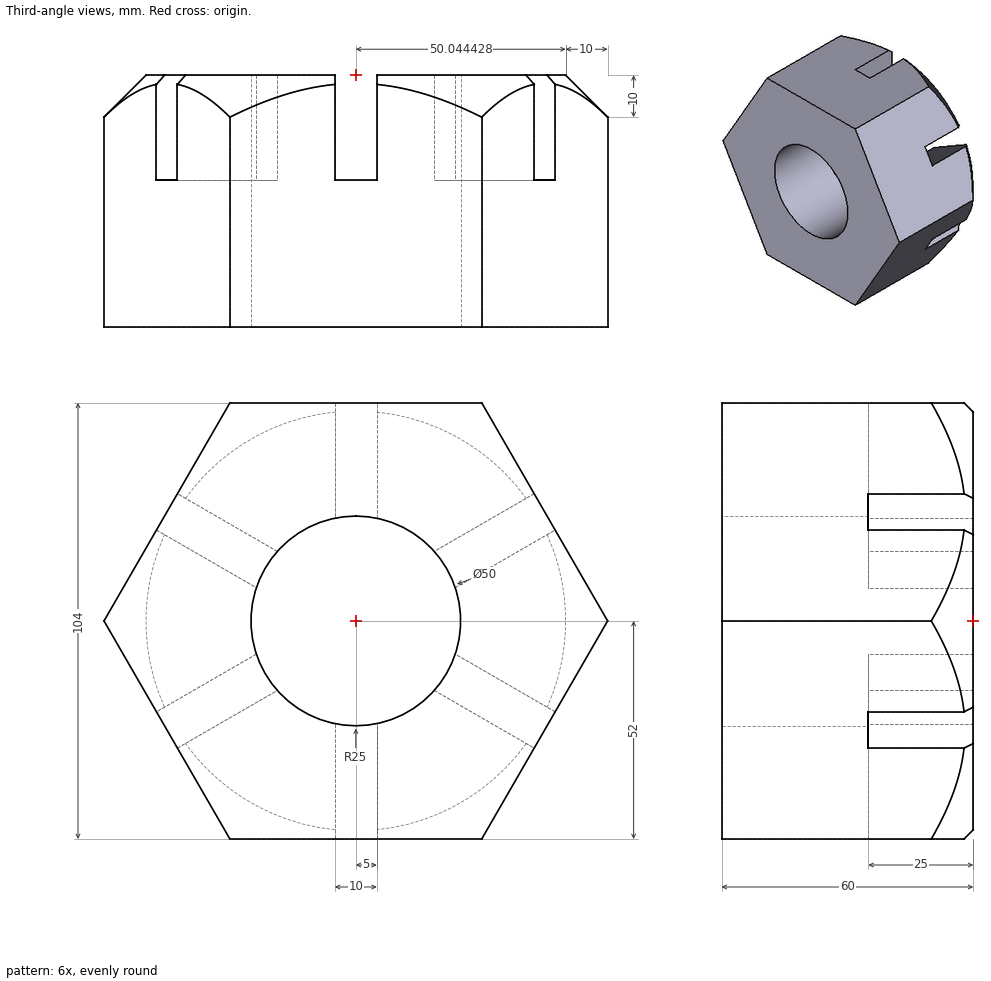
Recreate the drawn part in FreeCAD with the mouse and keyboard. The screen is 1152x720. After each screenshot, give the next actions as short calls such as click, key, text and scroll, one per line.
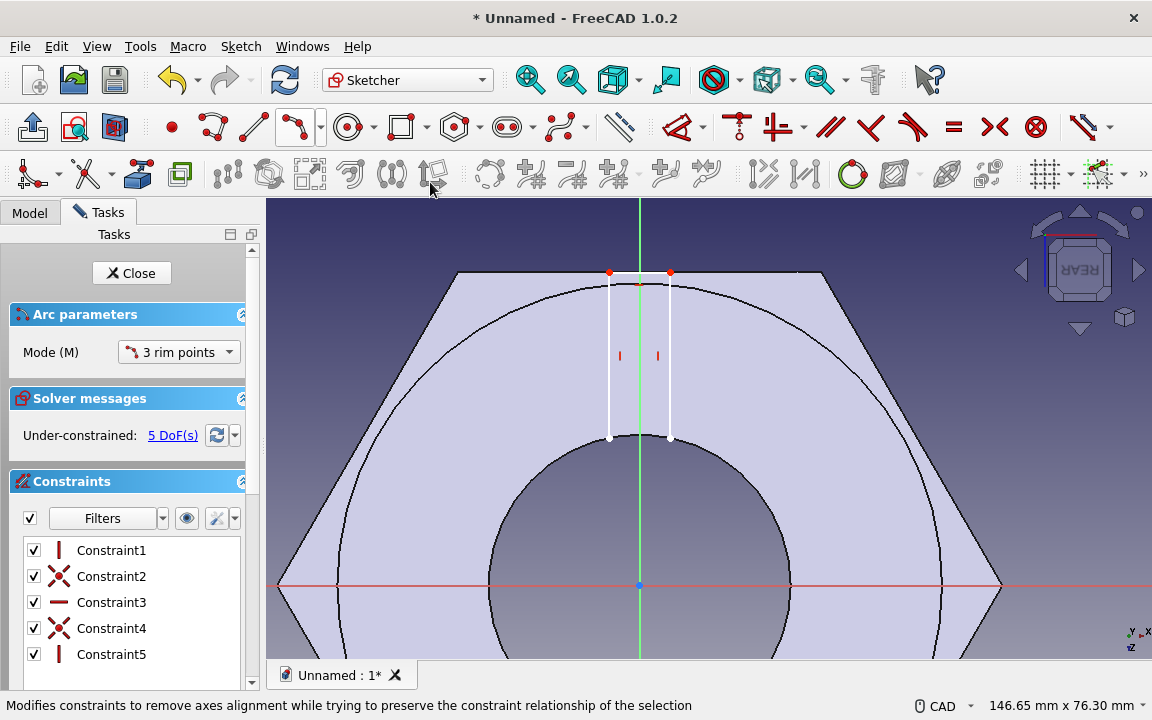
click(609, 439)
click(670, 439)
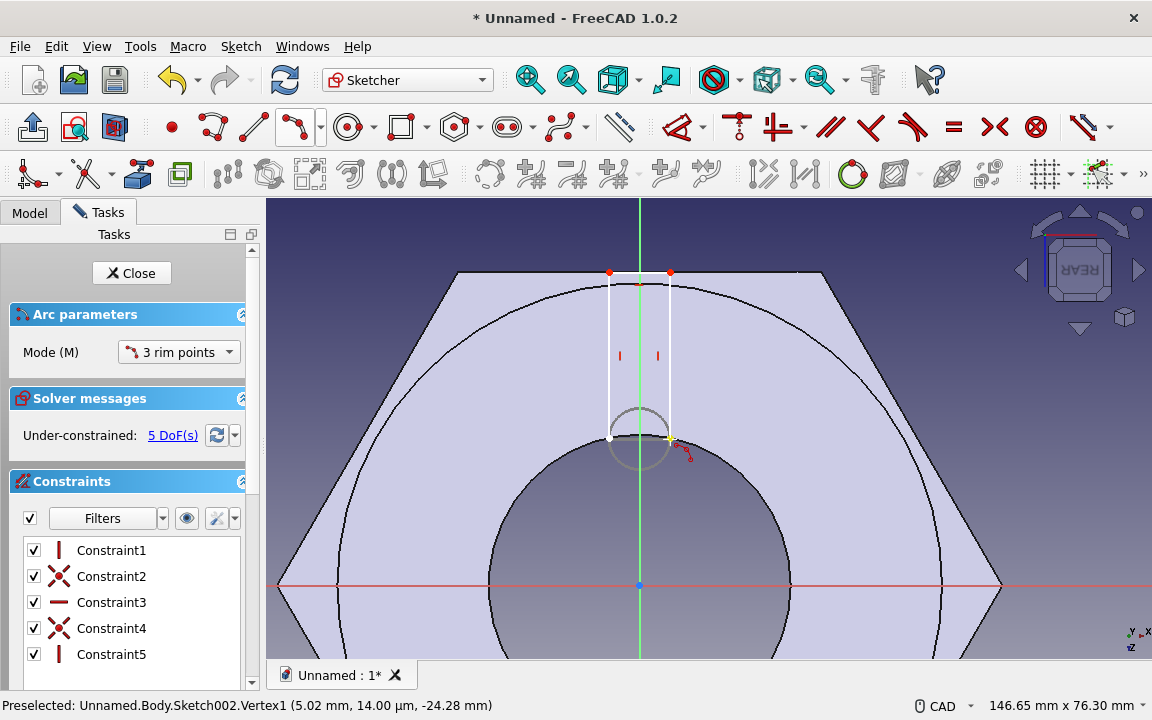
scroll(646, 435, up, 9)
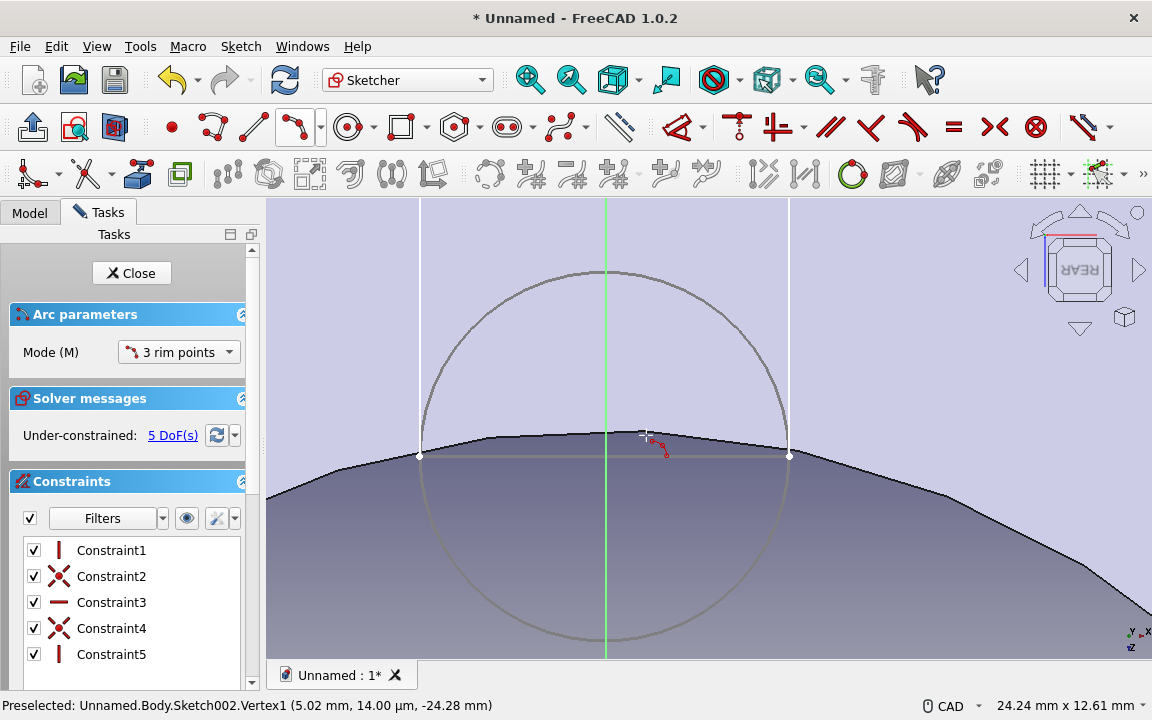
click(642, 431)
key(Escape)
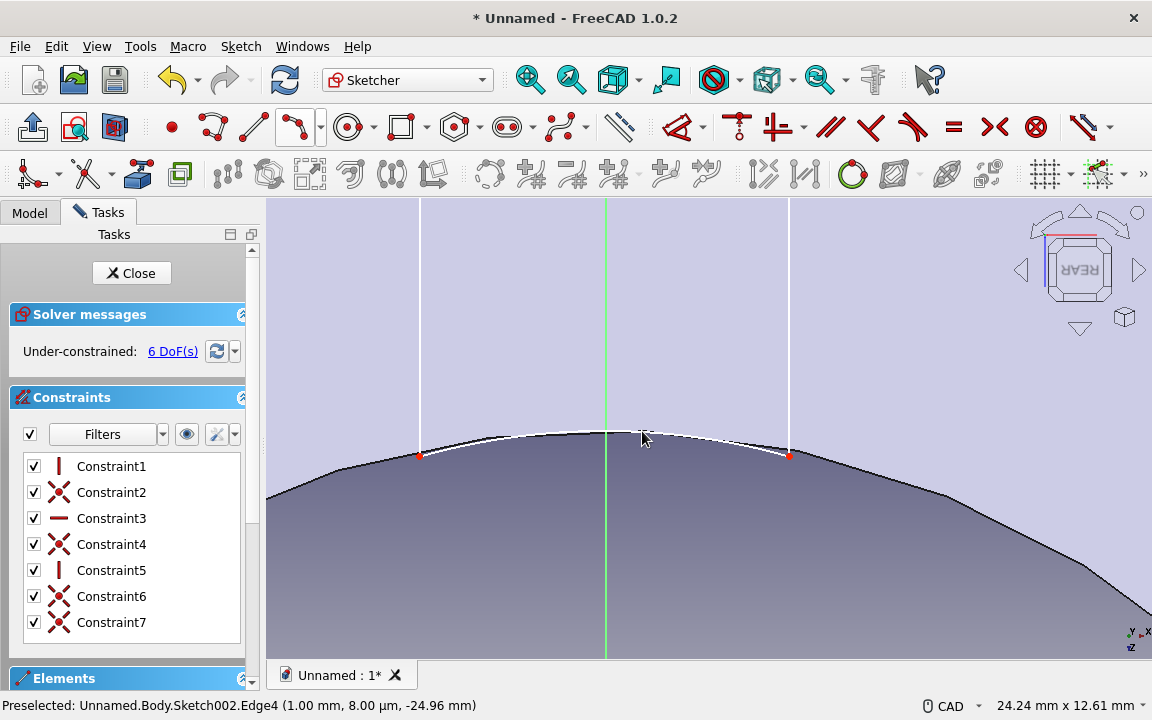
scroll(647, 435, down, 9)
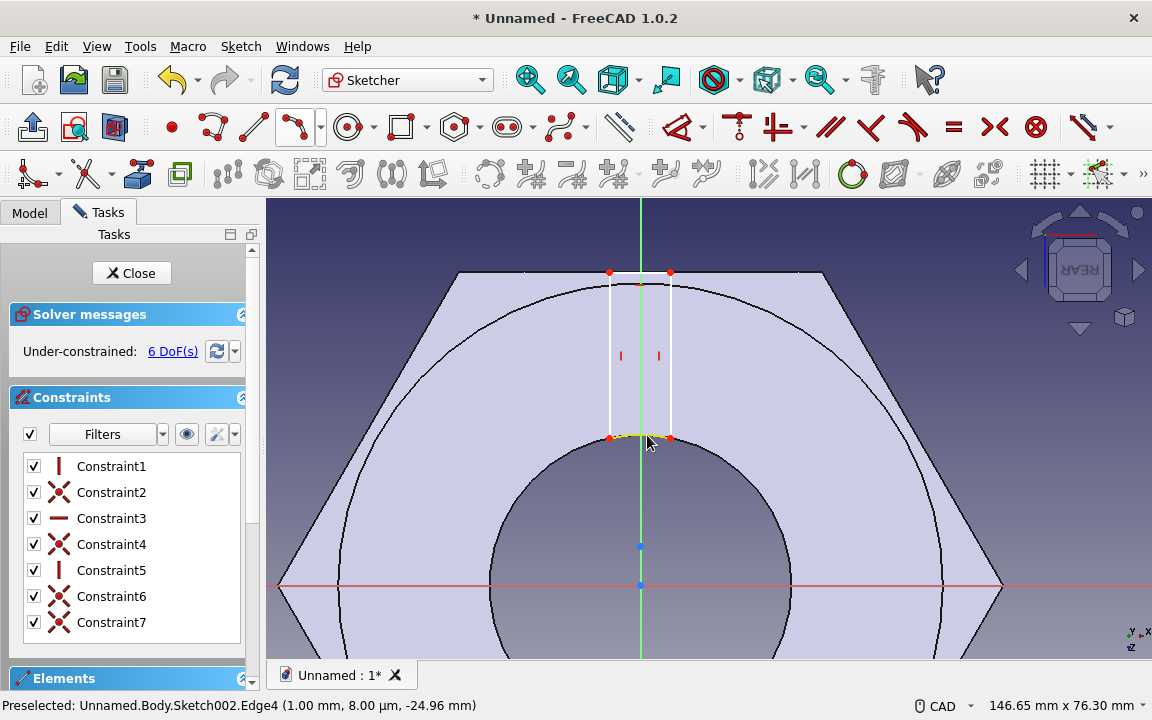
drag(630, 537, 651, 596)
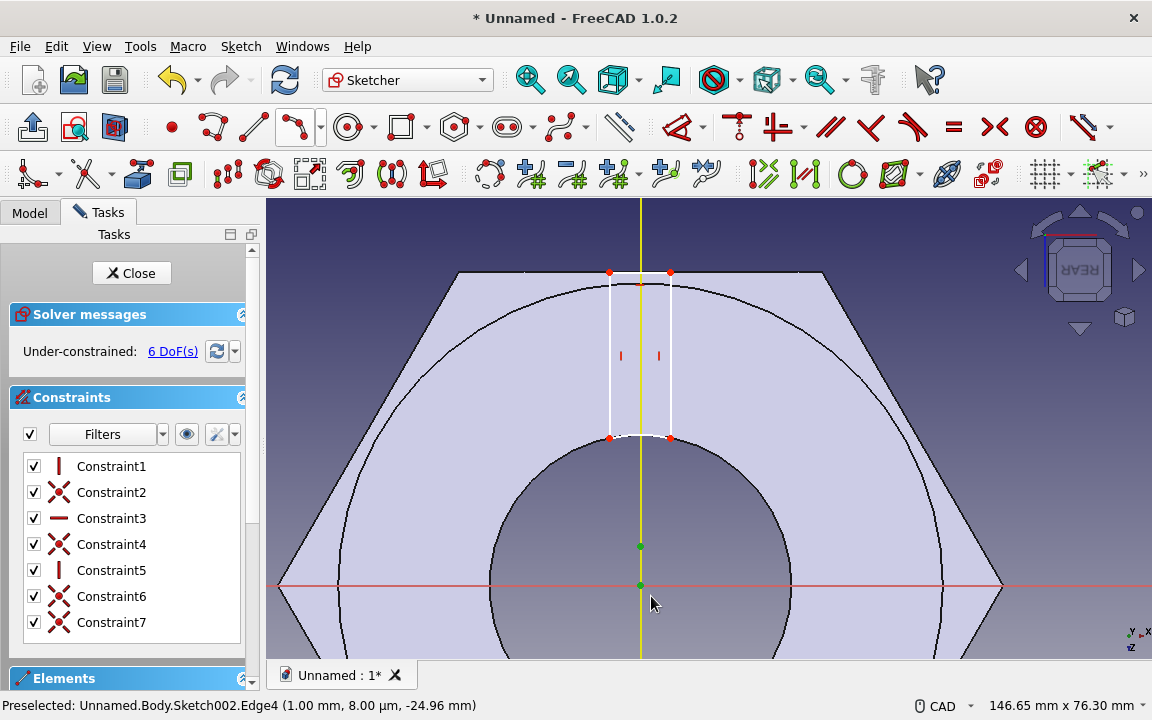
click(737, 128)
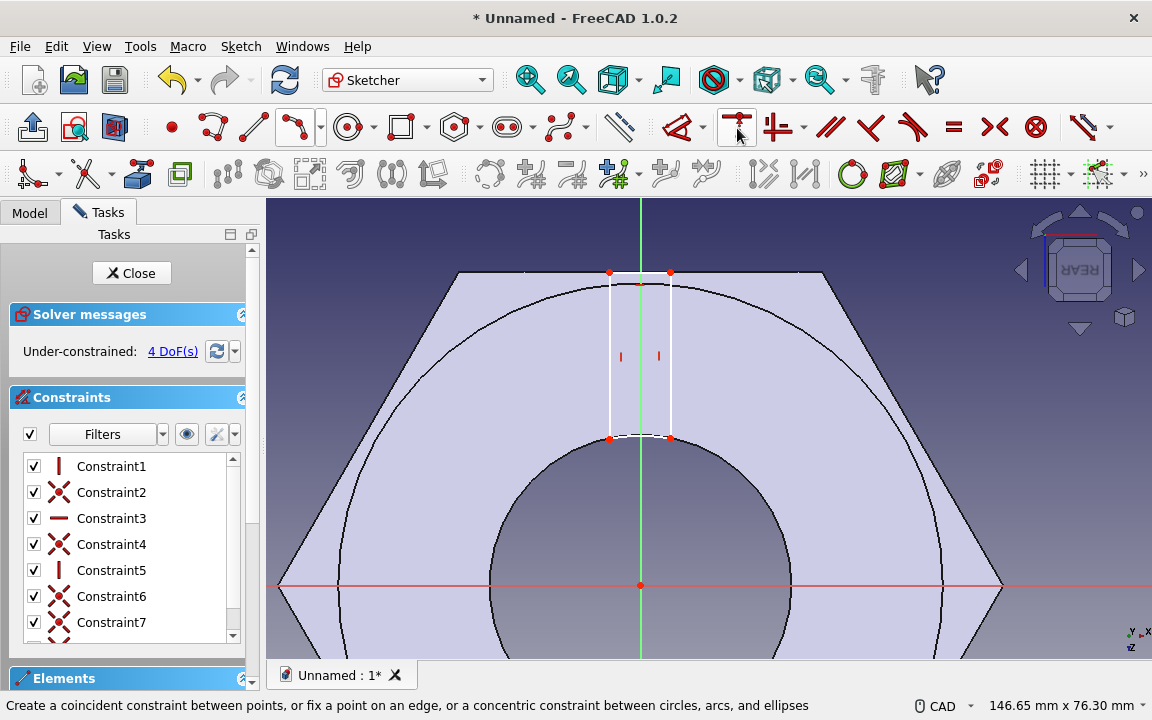
click(676, 128)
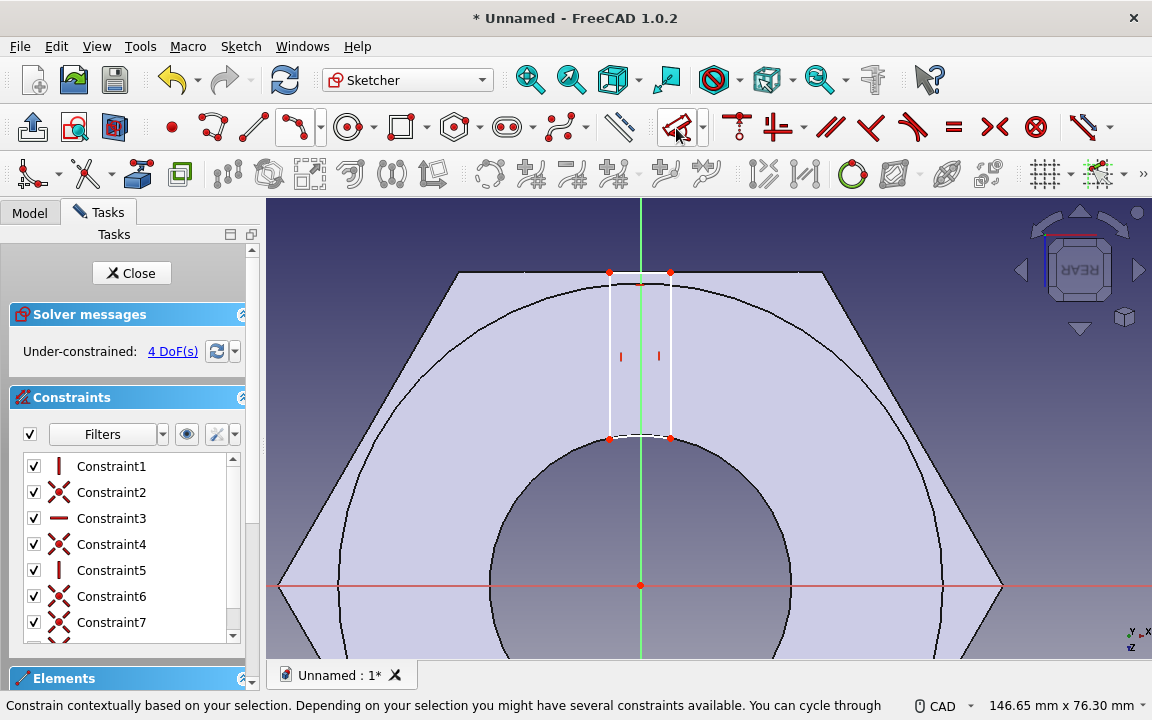
click(653, 436)
click(656, 404)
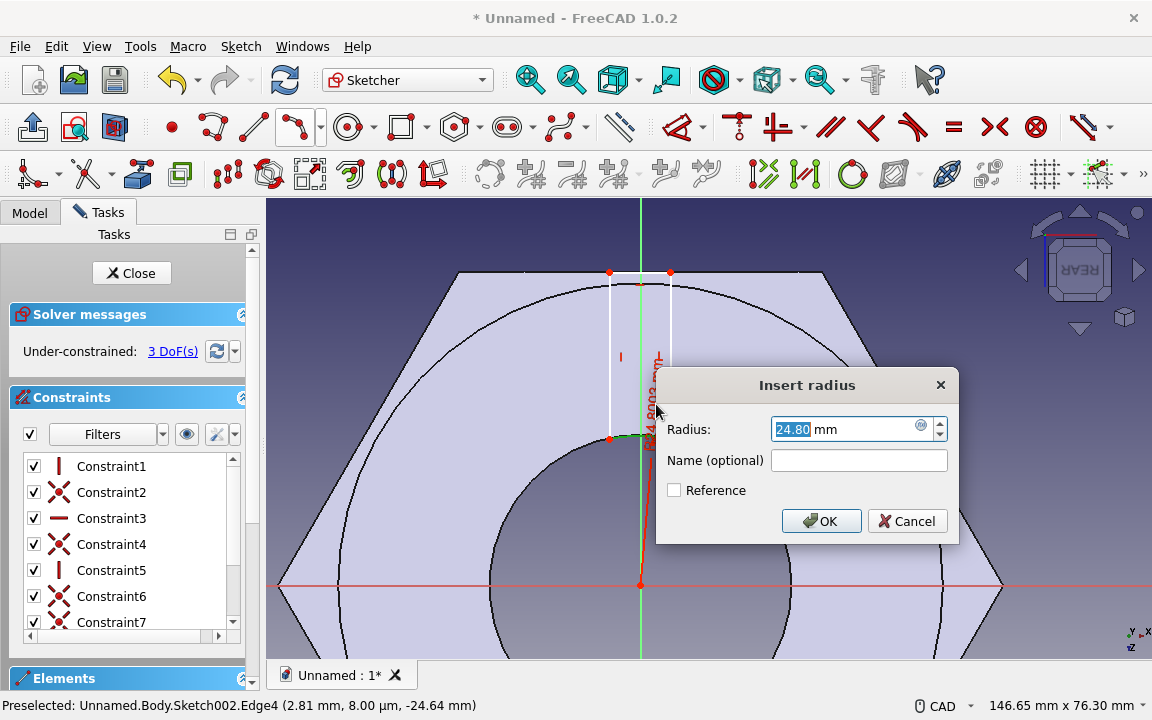
text(25)
key(Return)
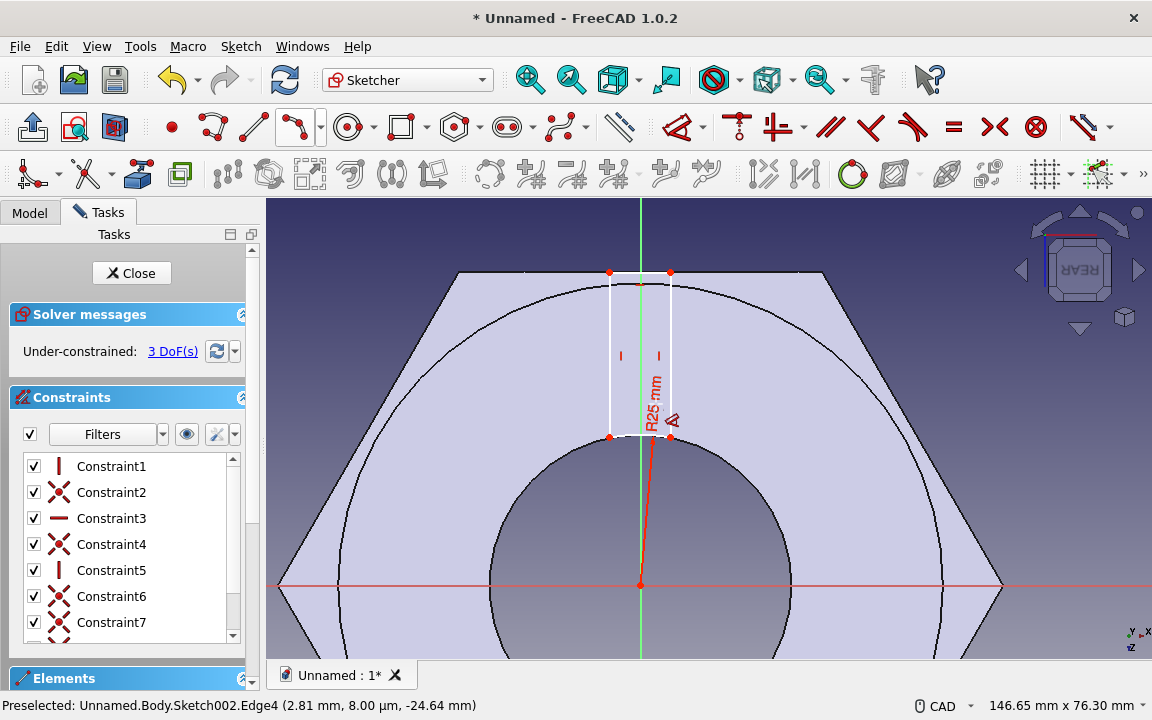
click(653, 273)
click(626, 239)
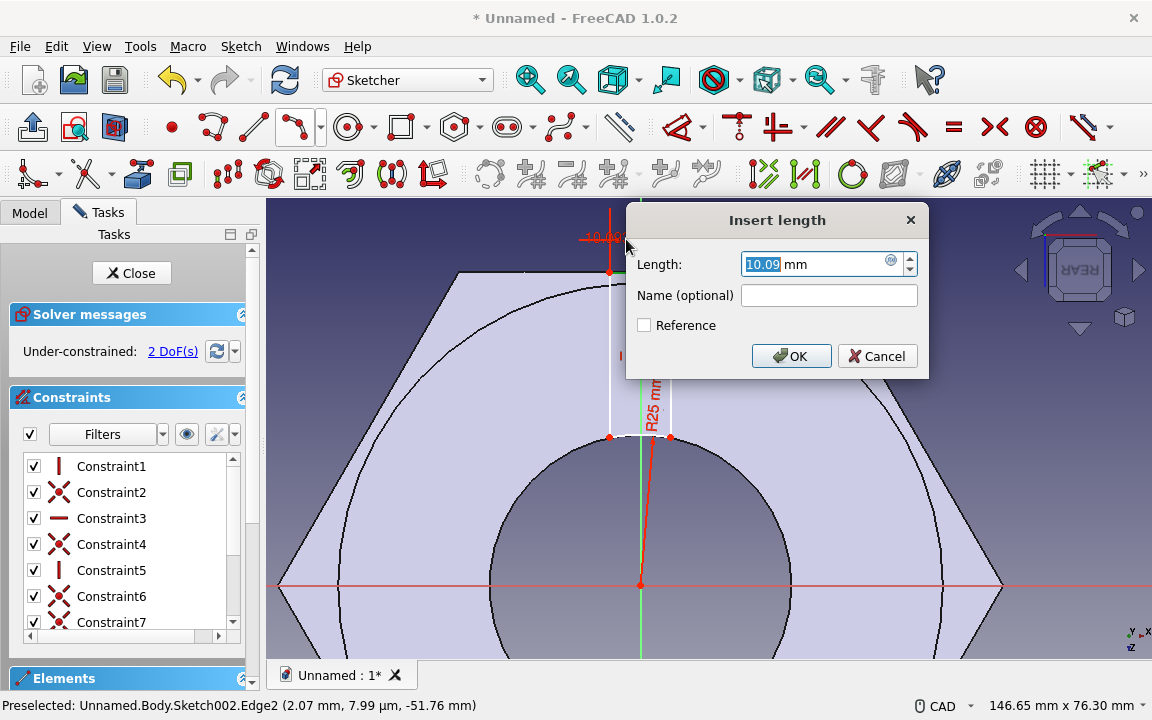
text(10)
key(Return)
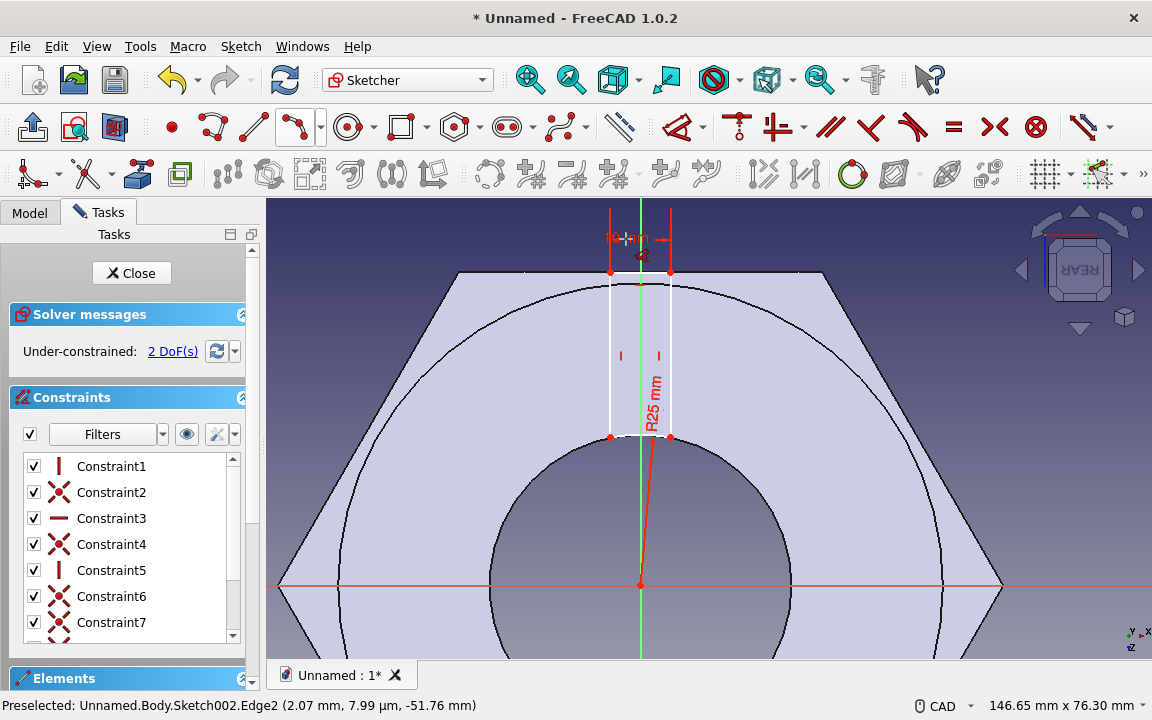
scroll(671, 438, up, 2)